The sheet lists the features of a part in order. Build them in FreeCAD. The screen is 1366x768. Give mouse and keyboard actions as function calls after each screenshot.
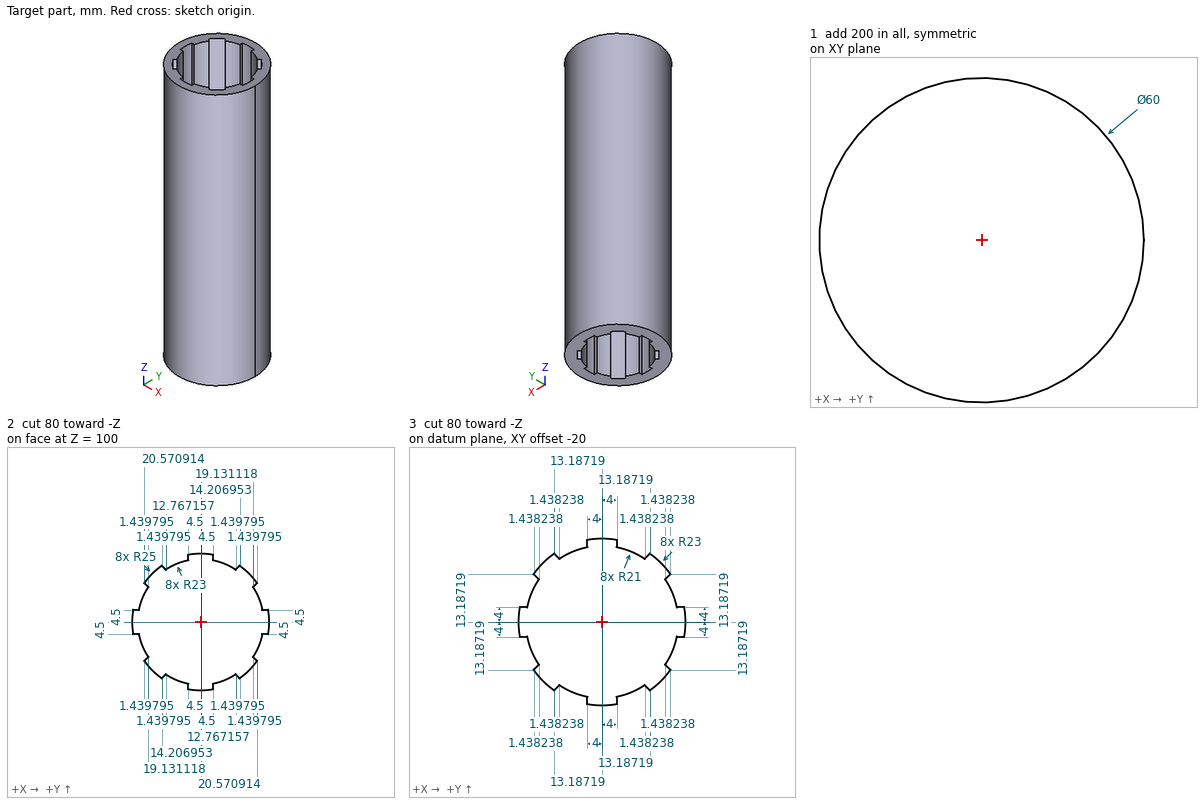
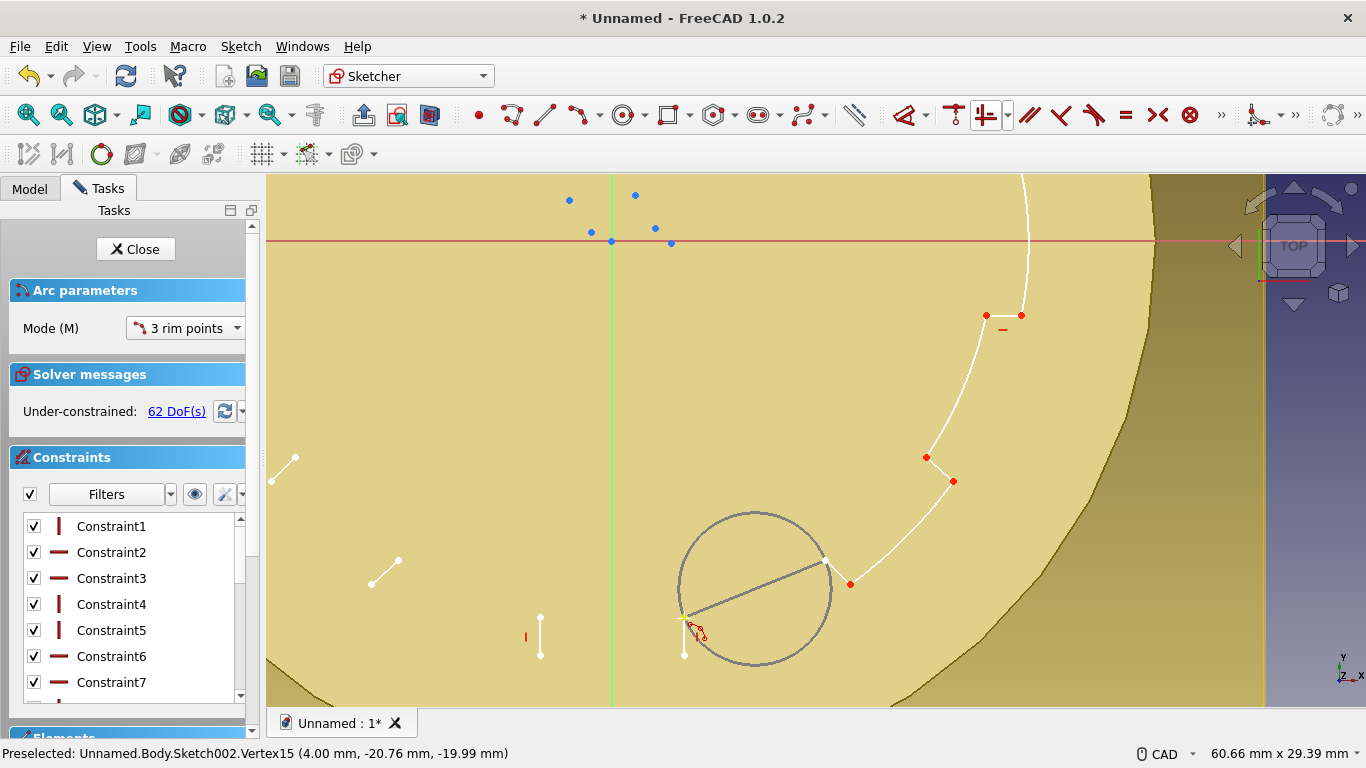
scroll(758, 593, up, 4)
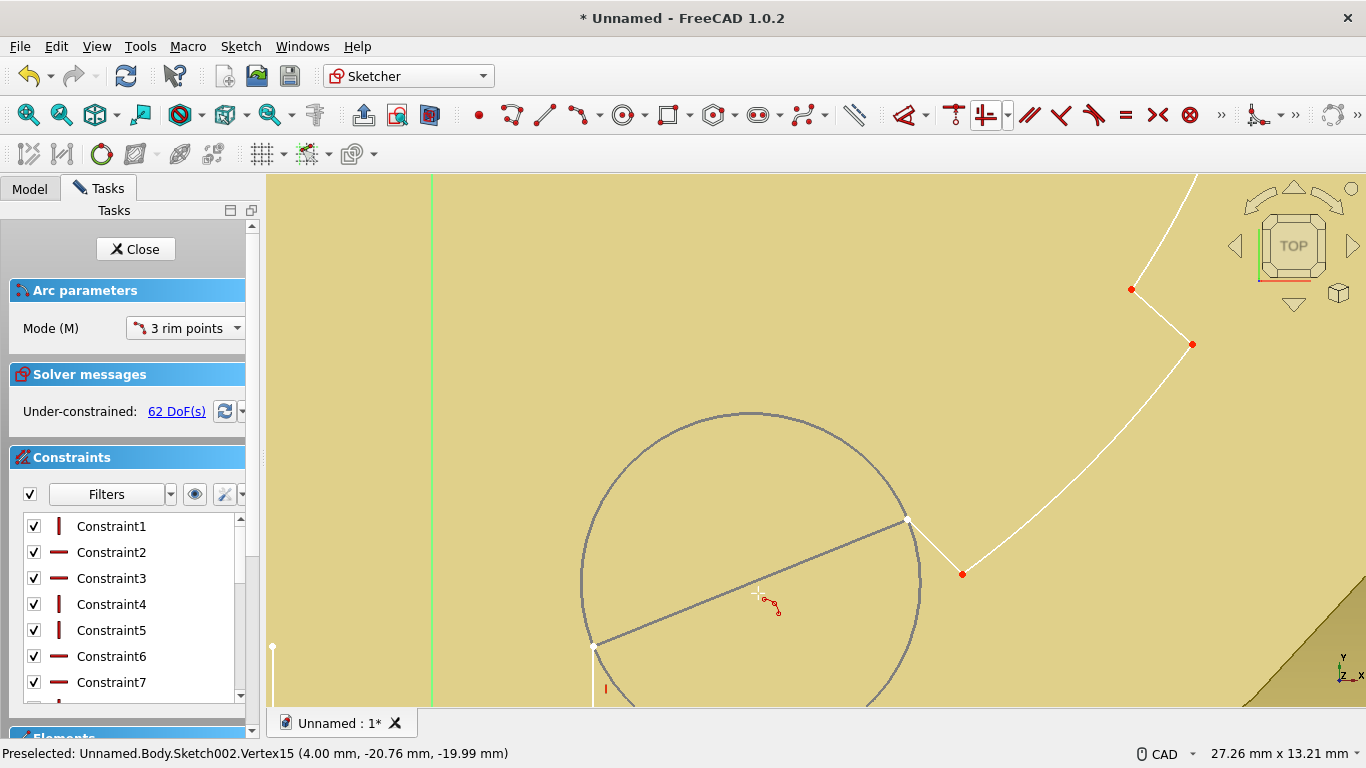
click(756, 592)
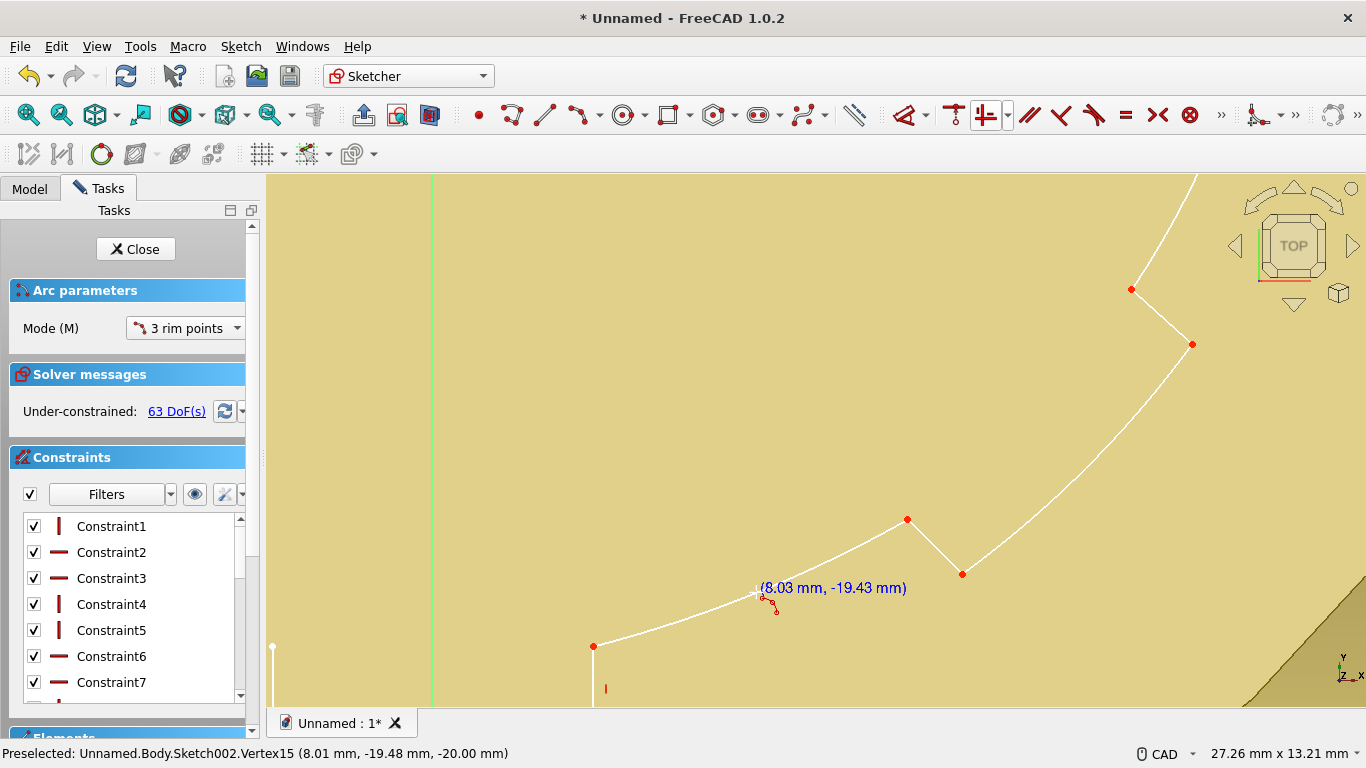
scroll(810, 566, down, 9)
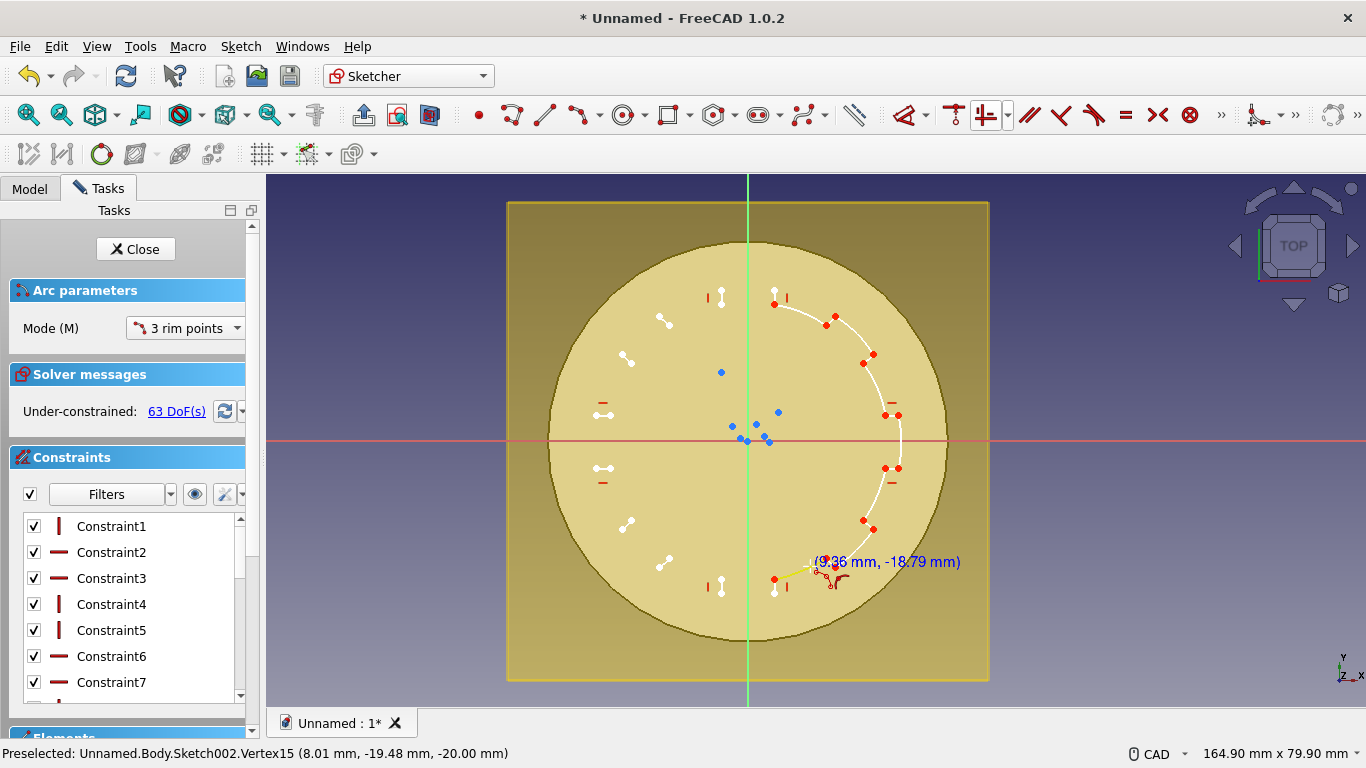
scroll(775, 593, up, 5)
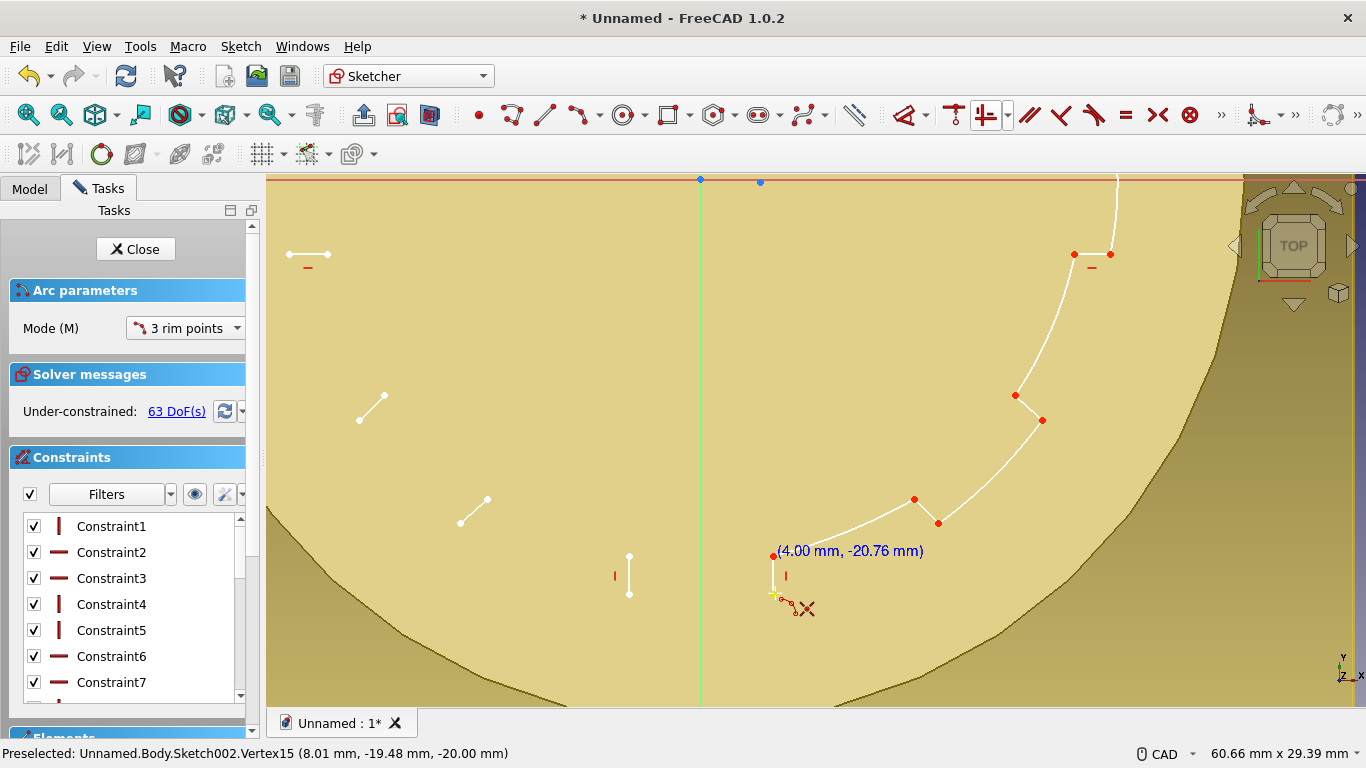
click(773, 594)
click(629, 594)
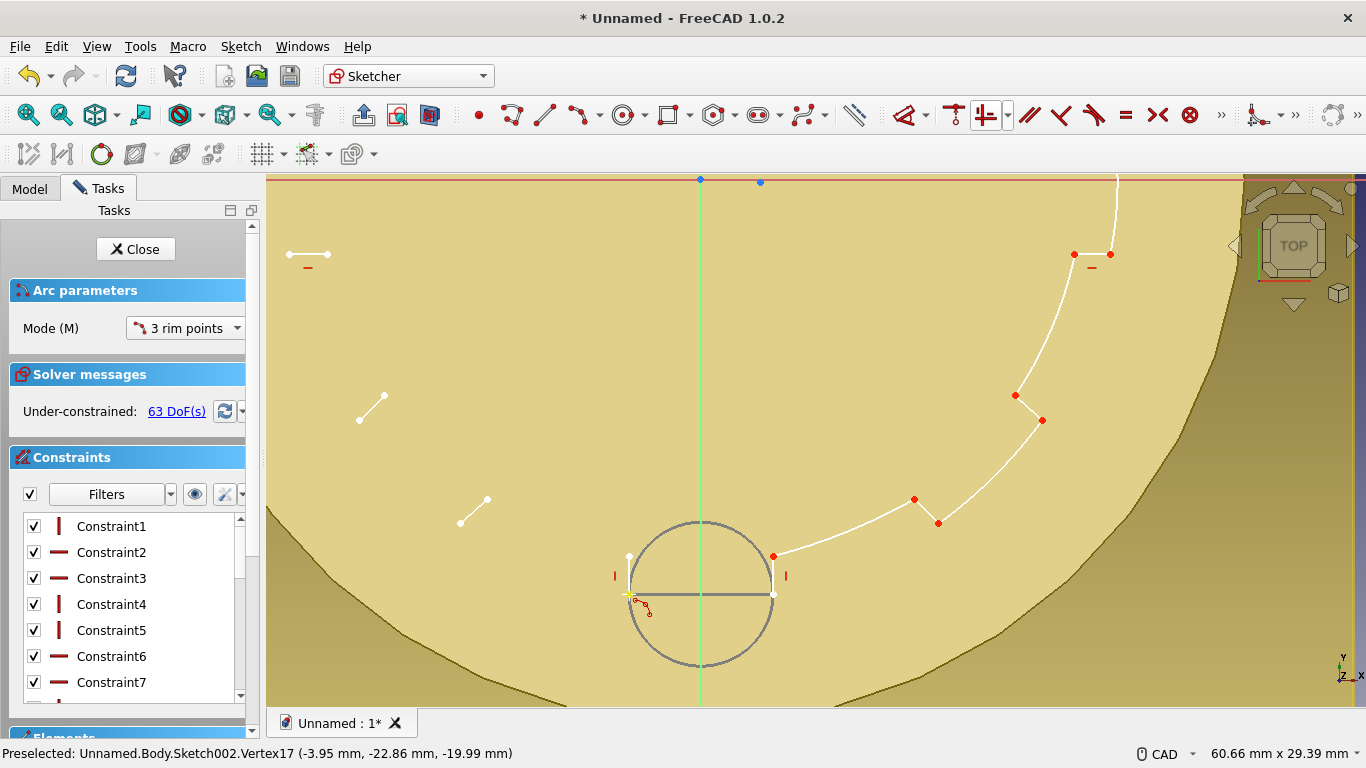
scroll(686, 596, up, 5)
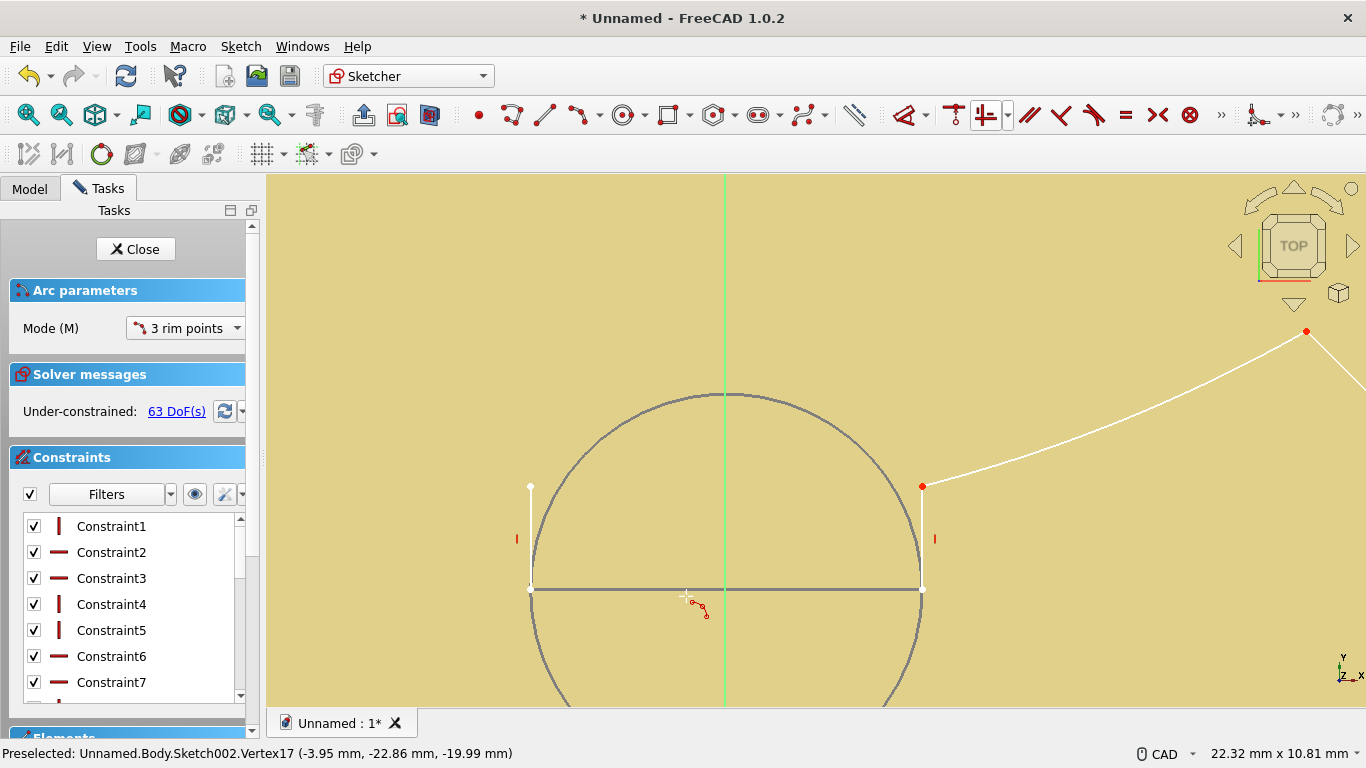
click(686, 596)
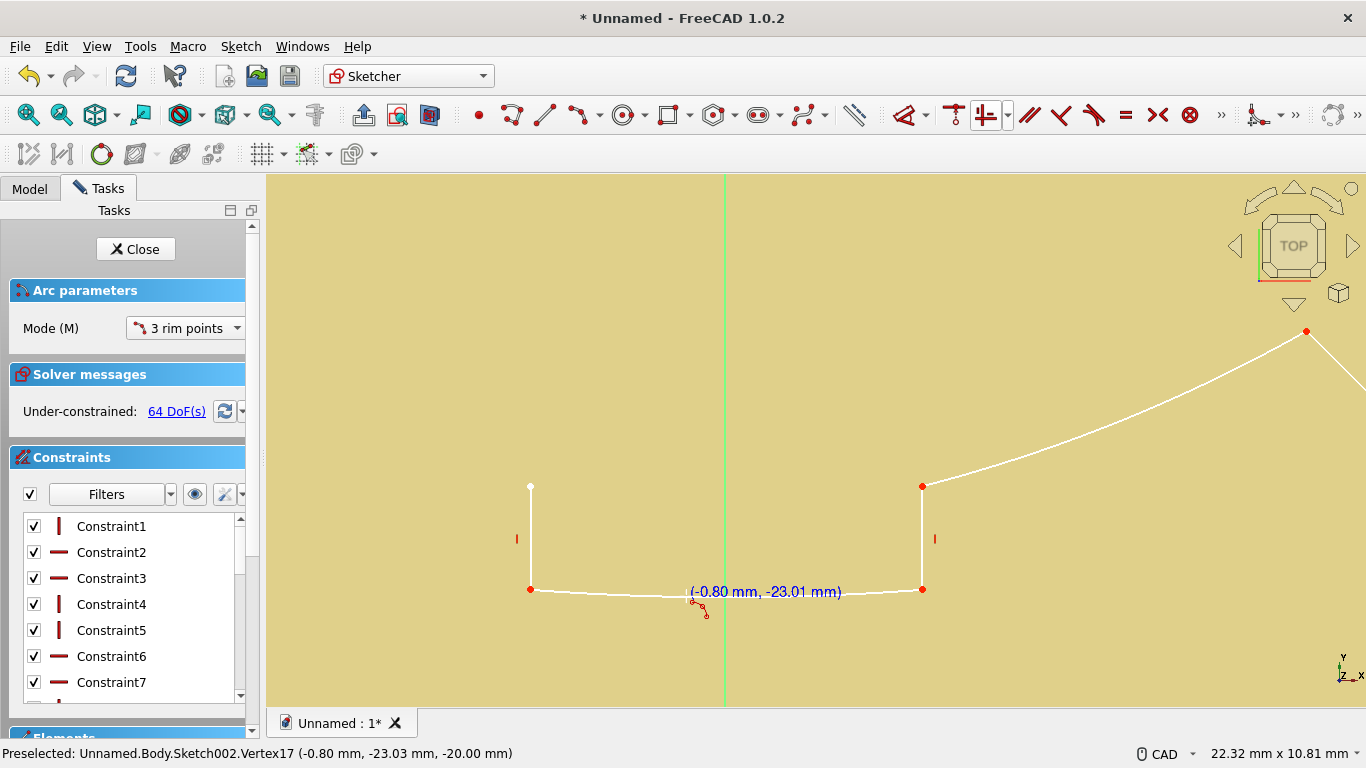
scroll(751, 594, down, 10)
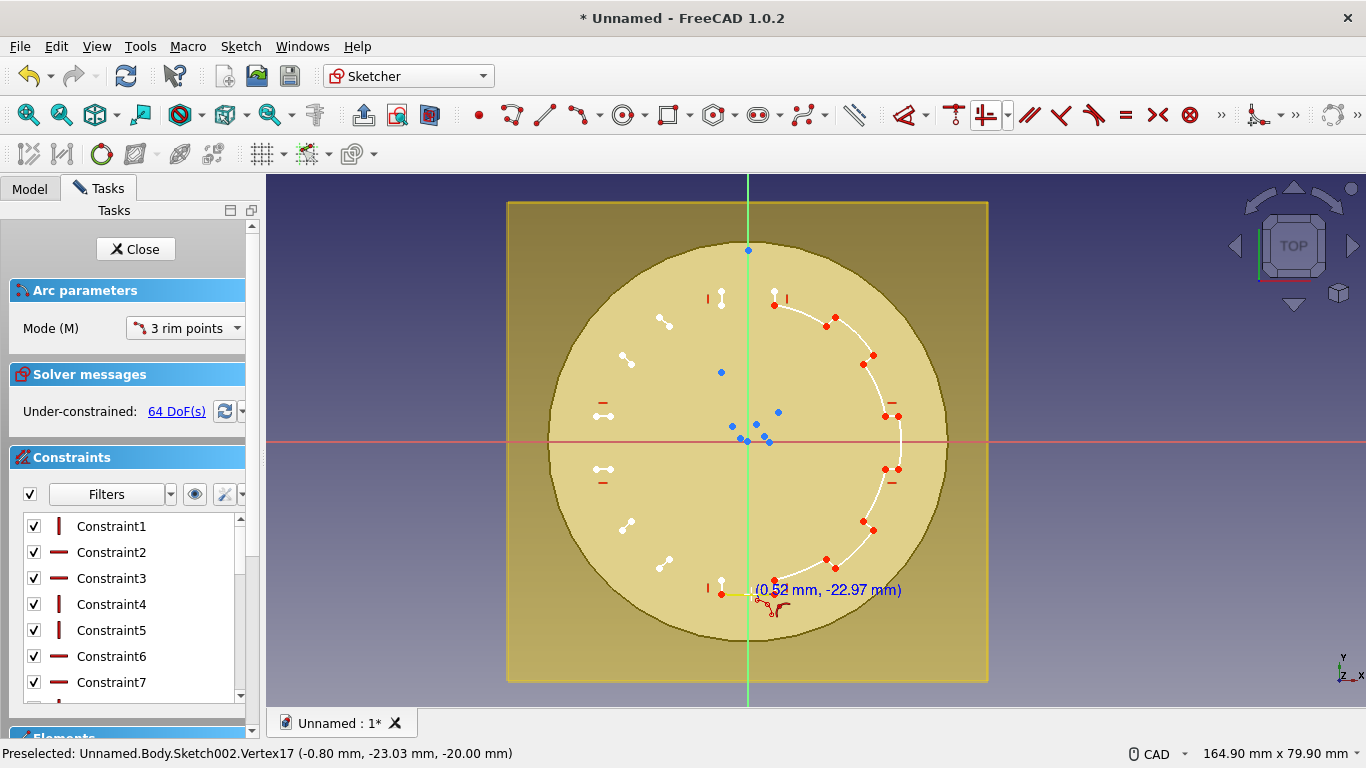
scroll(721, 579, up, 5)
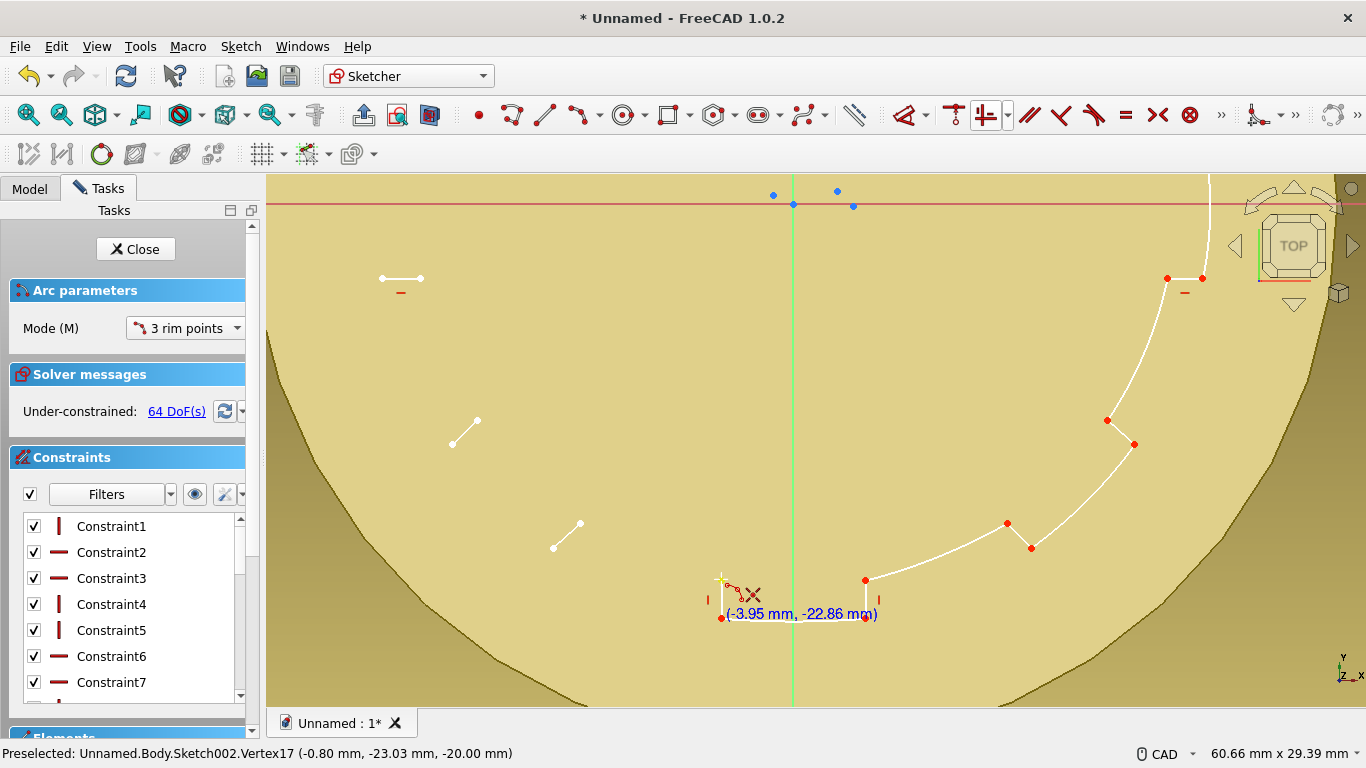
click(722, 581)
click(580, 524)